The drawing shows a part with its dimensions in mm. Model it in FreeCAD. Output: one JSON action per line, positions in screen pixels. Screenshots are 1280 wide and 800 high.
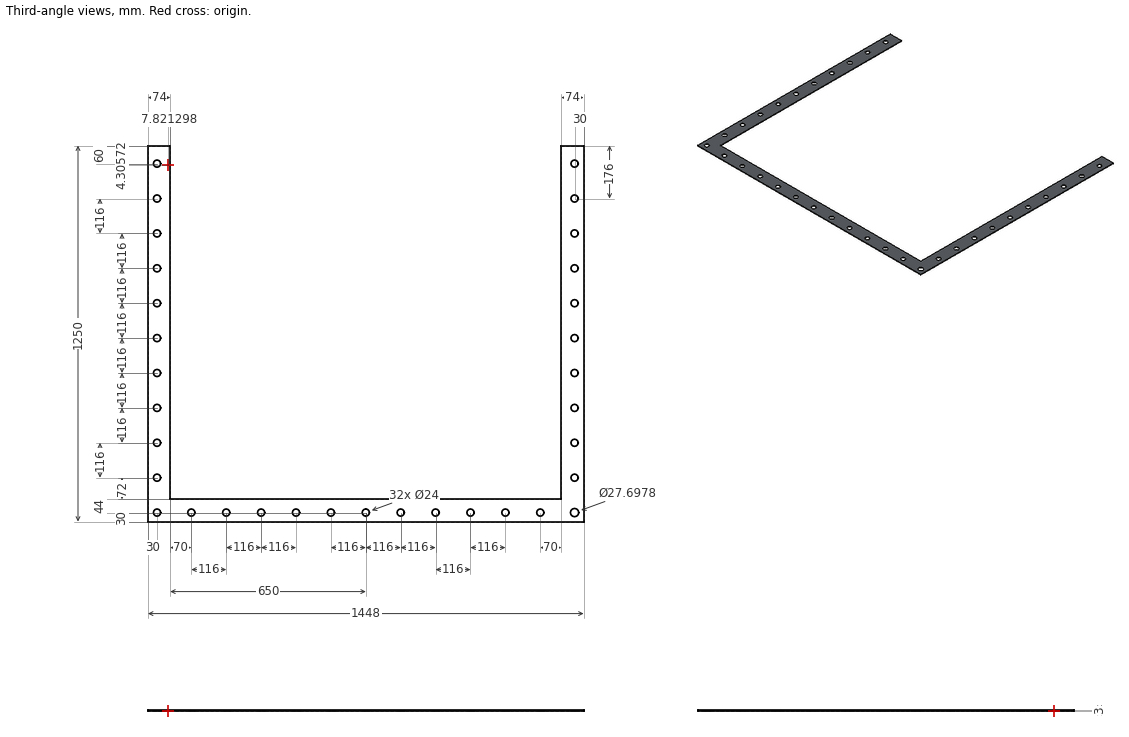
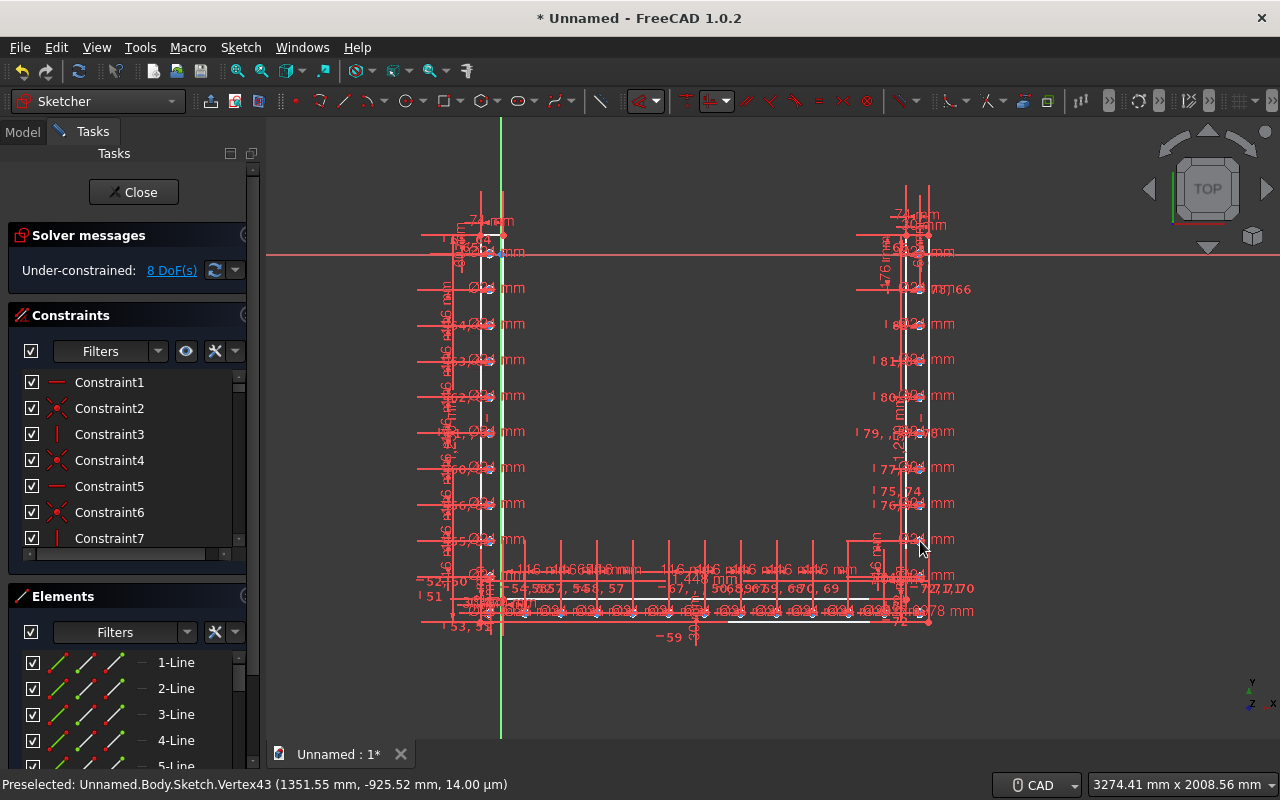
{"action": "left_click", "coordinate": [920, 541]}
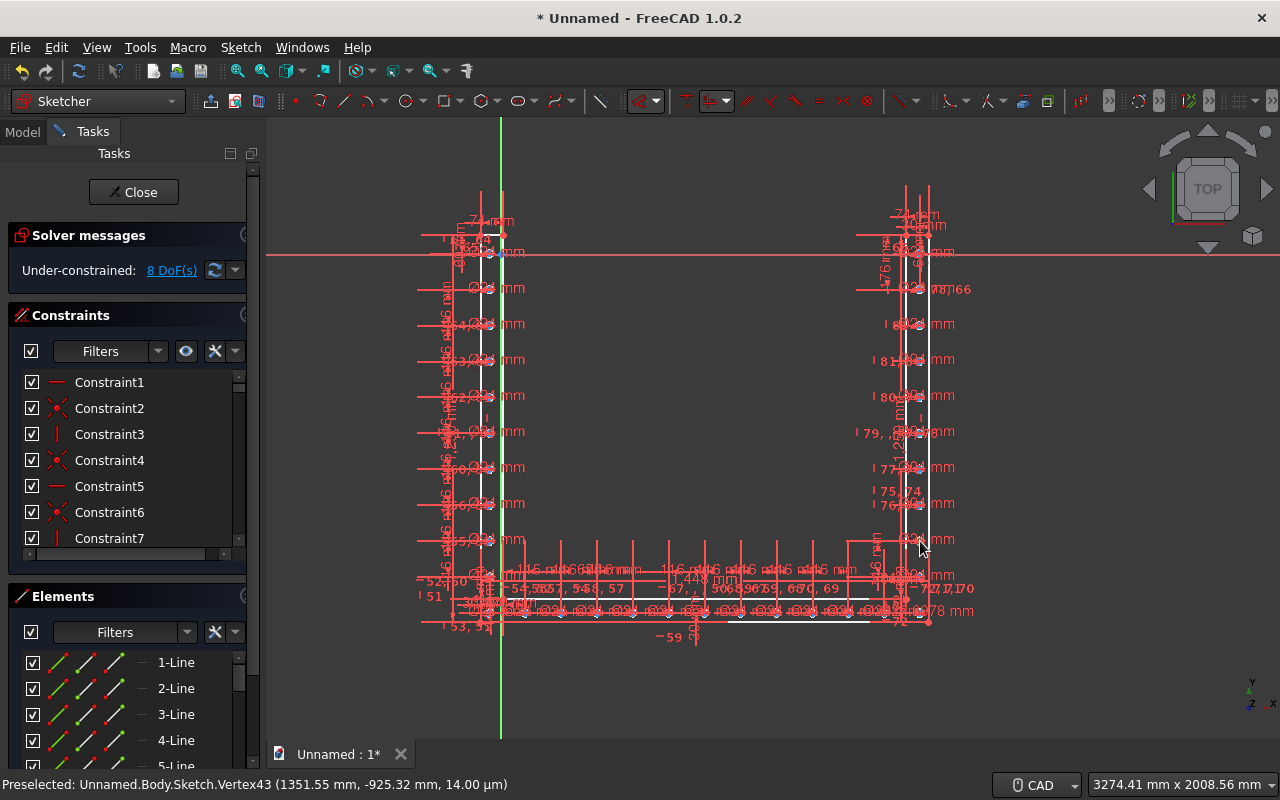
{"action": "left_click", "coordinate": [920, 505]}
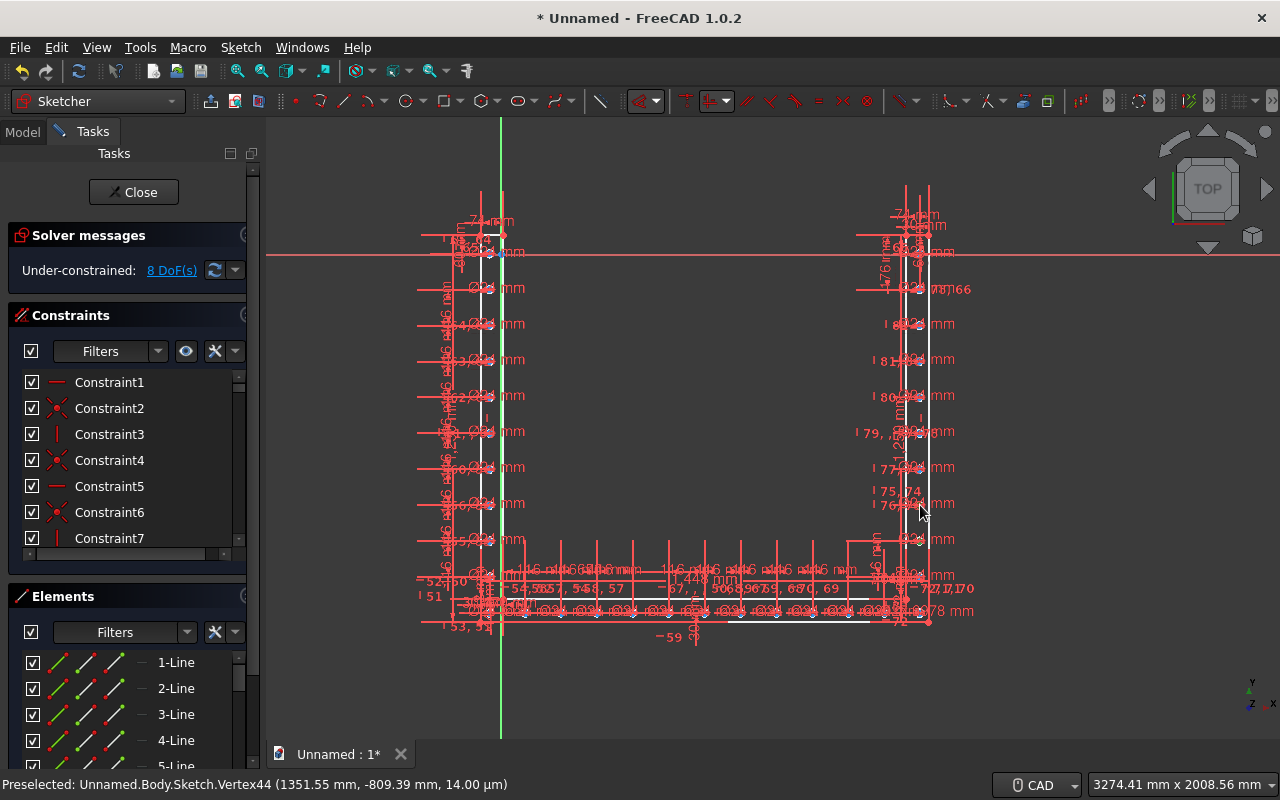
{"action": "left_click", "coordinate": [658, 102]}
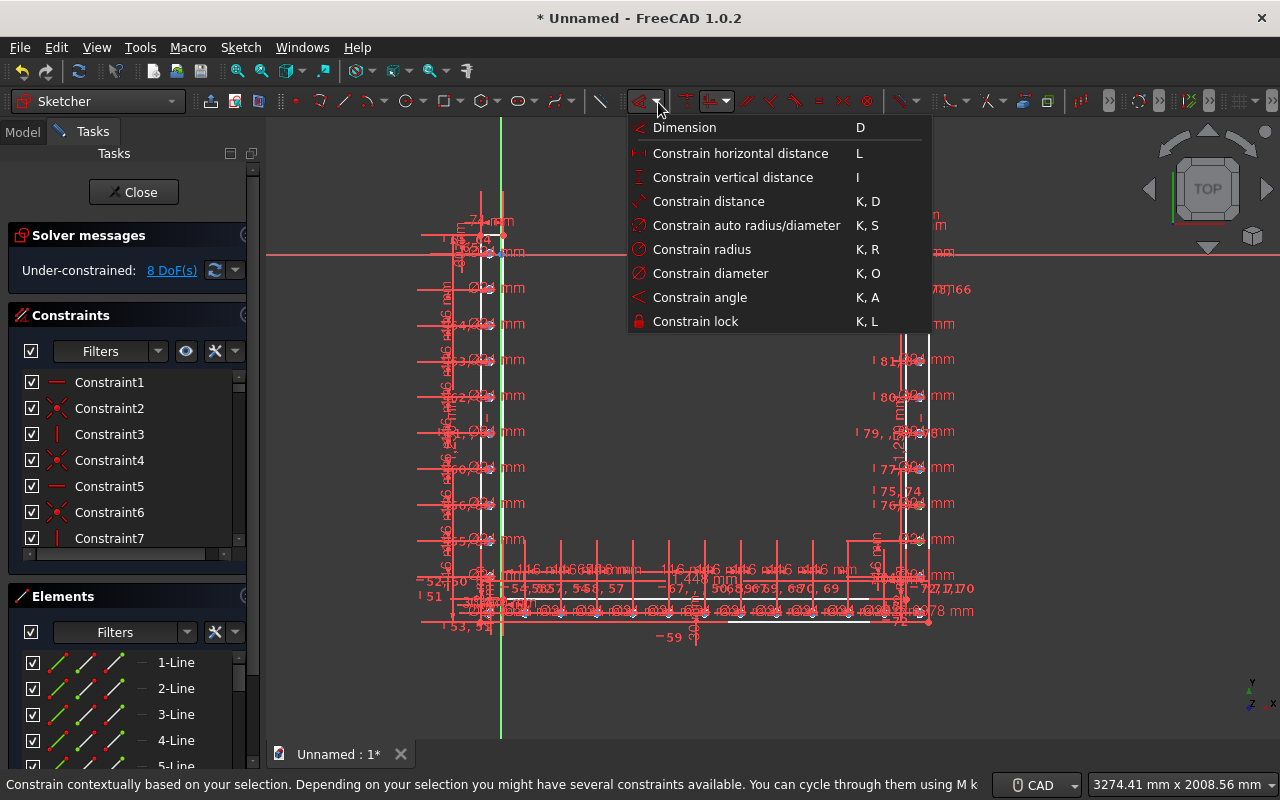
{"action": "left_click", "coordinate": [780, 177]}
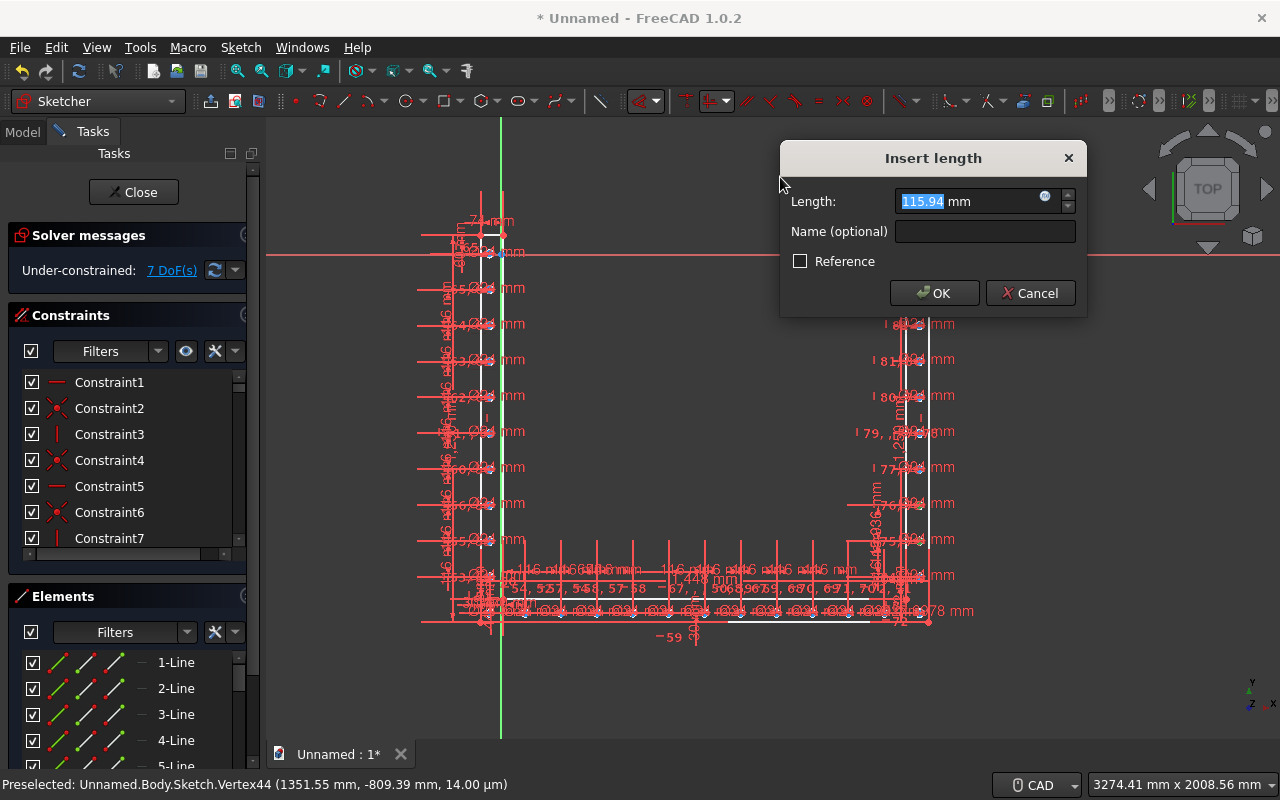
{"action": "type", "text": "116"}
{"action": "key", "text": "Return"}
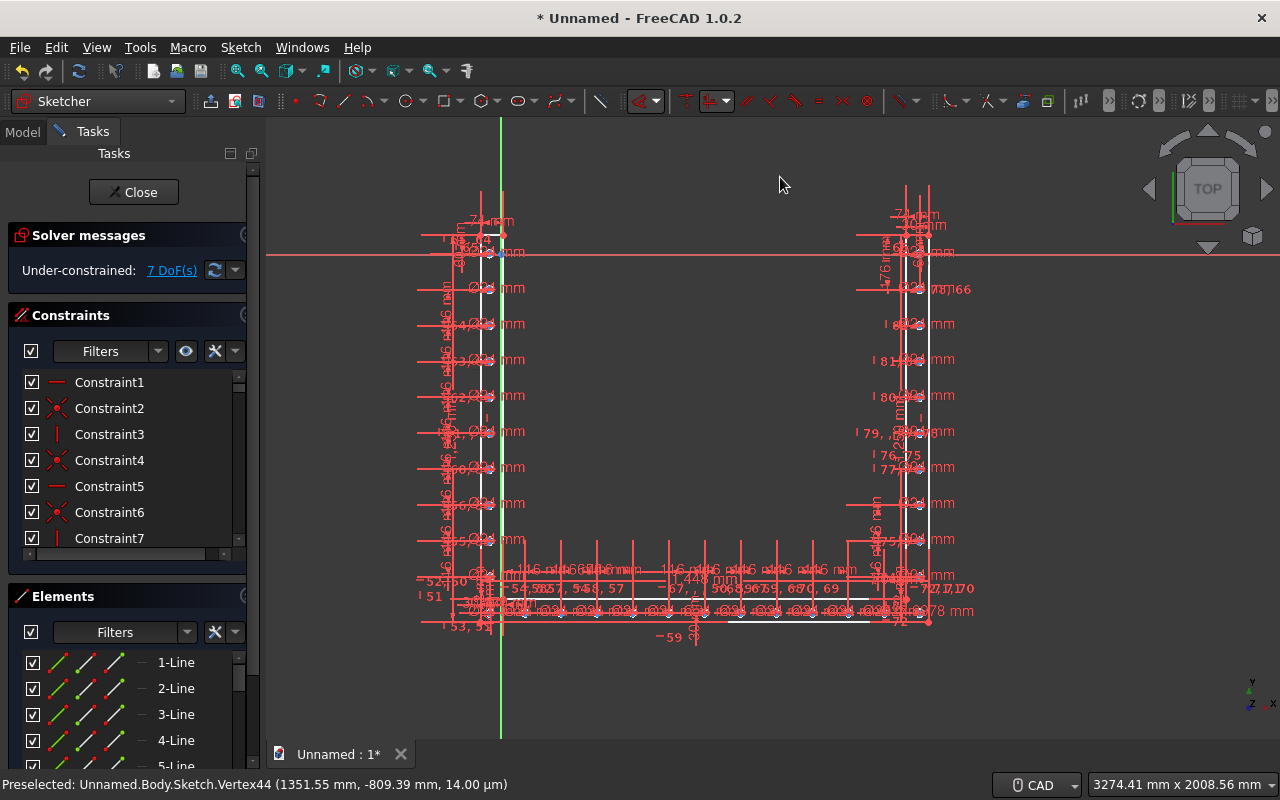
{"action": "left_click", "coordinate": [920, 505]}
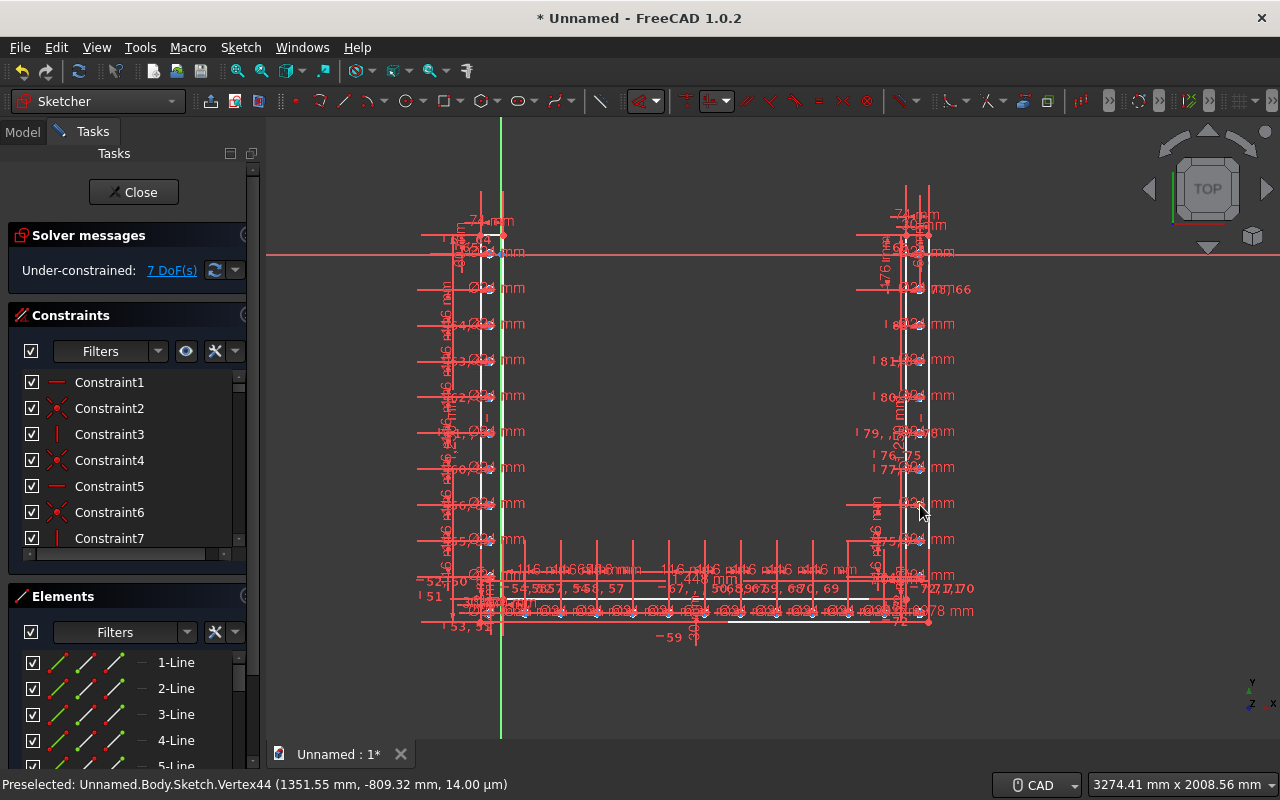
{"action": "left_click", "coordinate": [920, 469]}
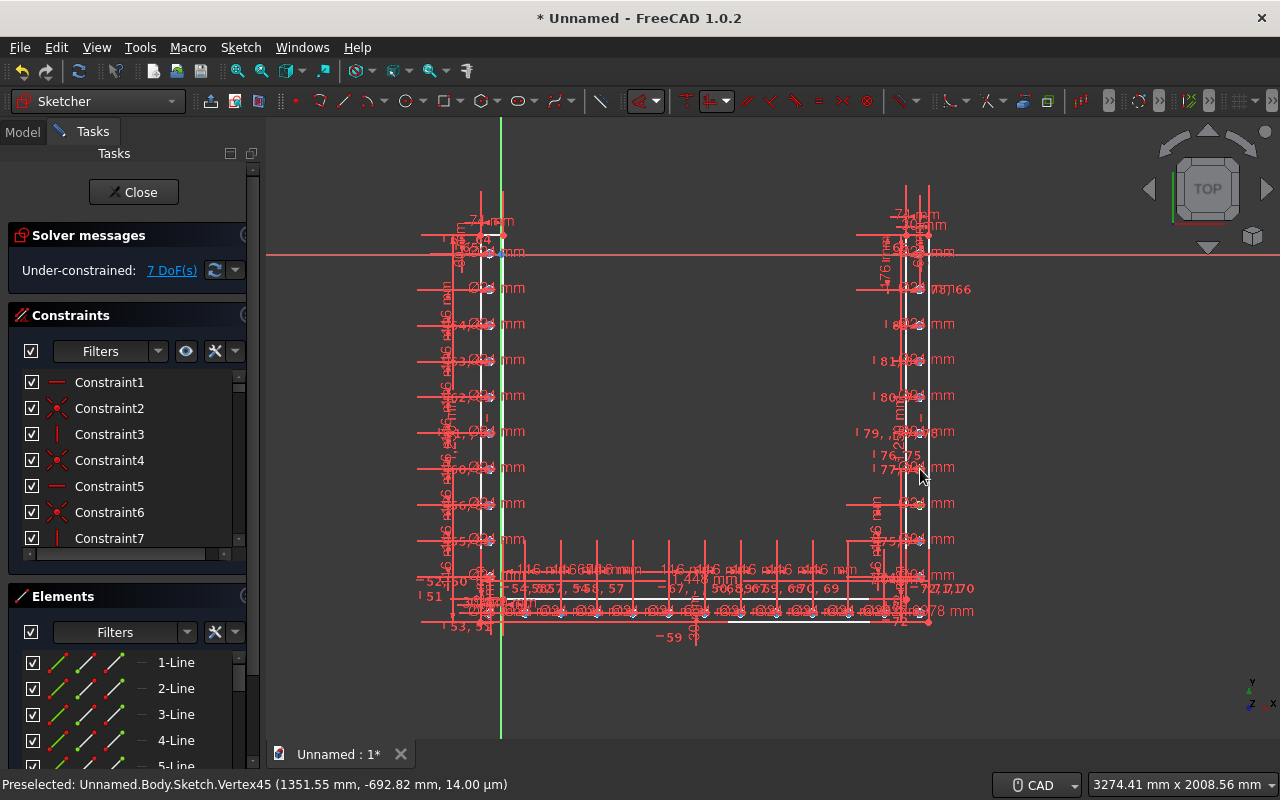
{"action": "left_click", "coordinate": [658, 102]}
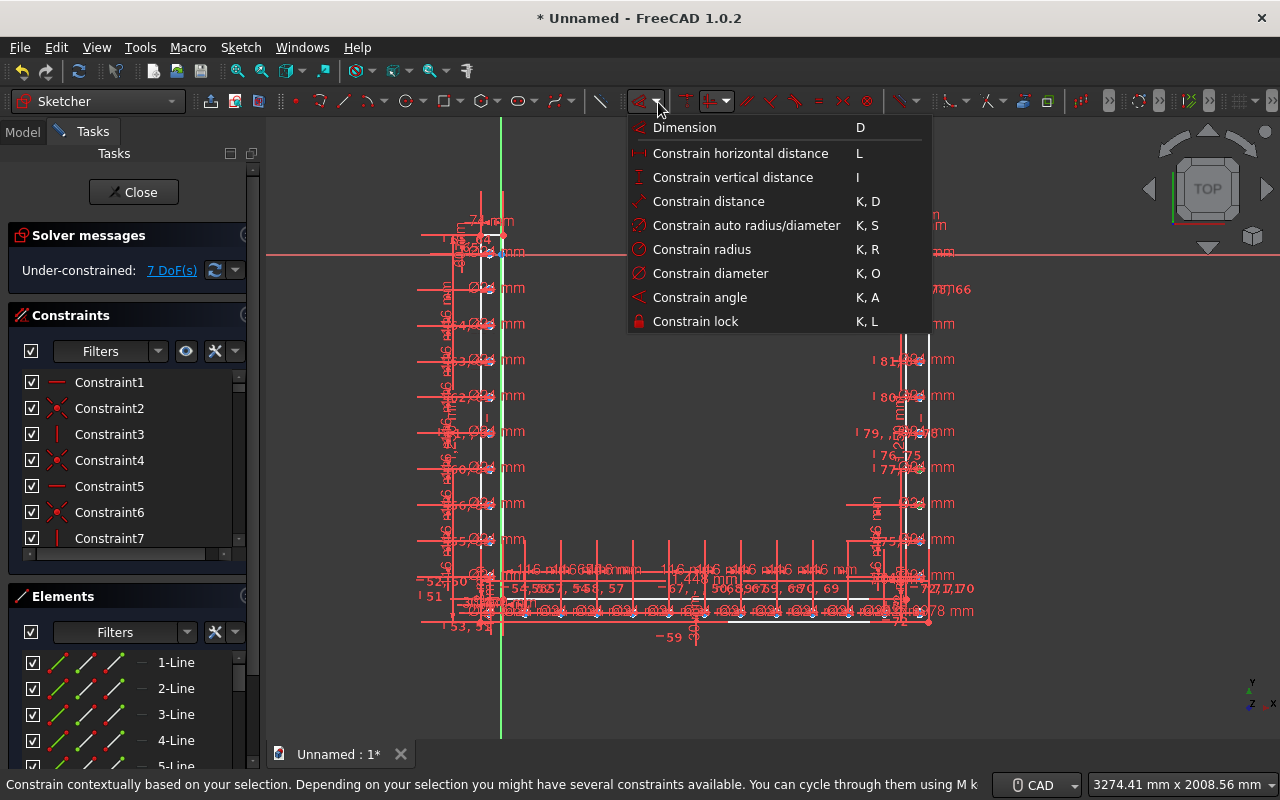
{"action": "left_click", "coordinate": [780, 177]}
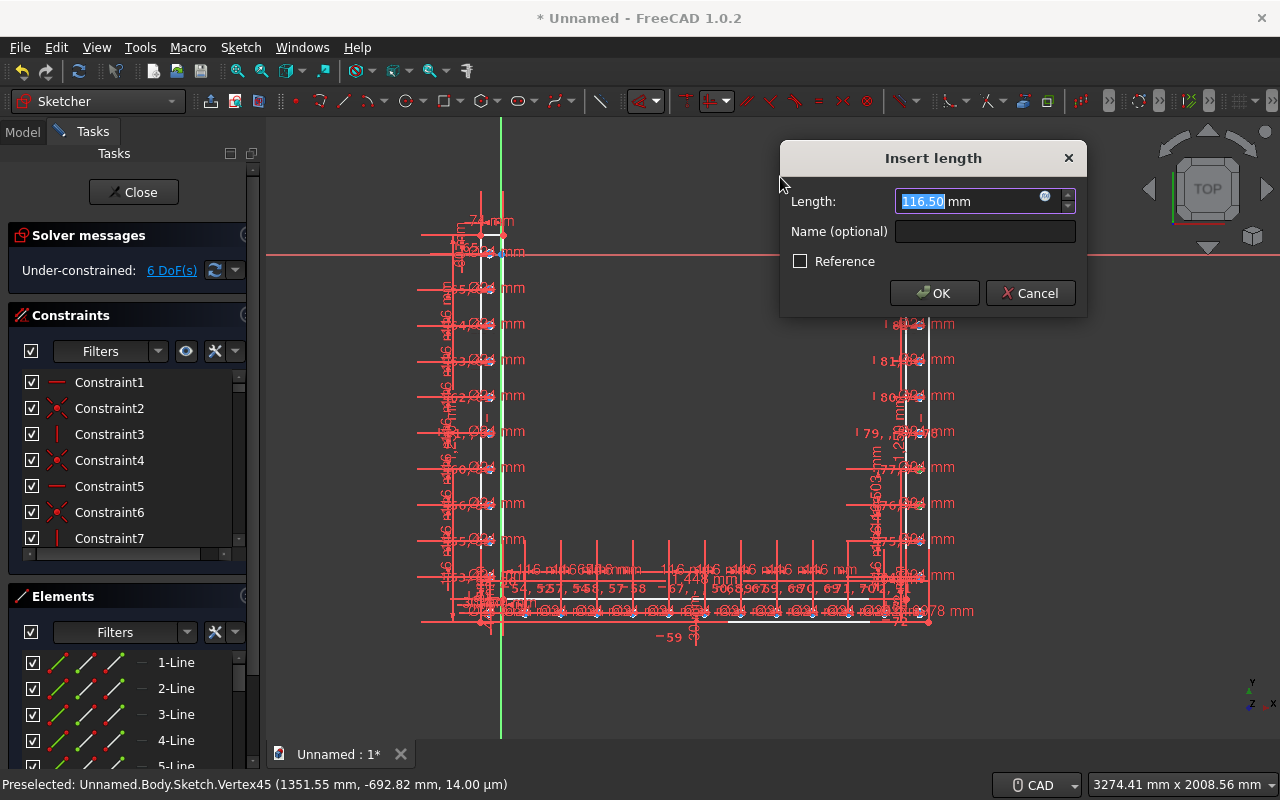
{"action": "type", "text": "116"}
{"action": "key", "text": "Return"}